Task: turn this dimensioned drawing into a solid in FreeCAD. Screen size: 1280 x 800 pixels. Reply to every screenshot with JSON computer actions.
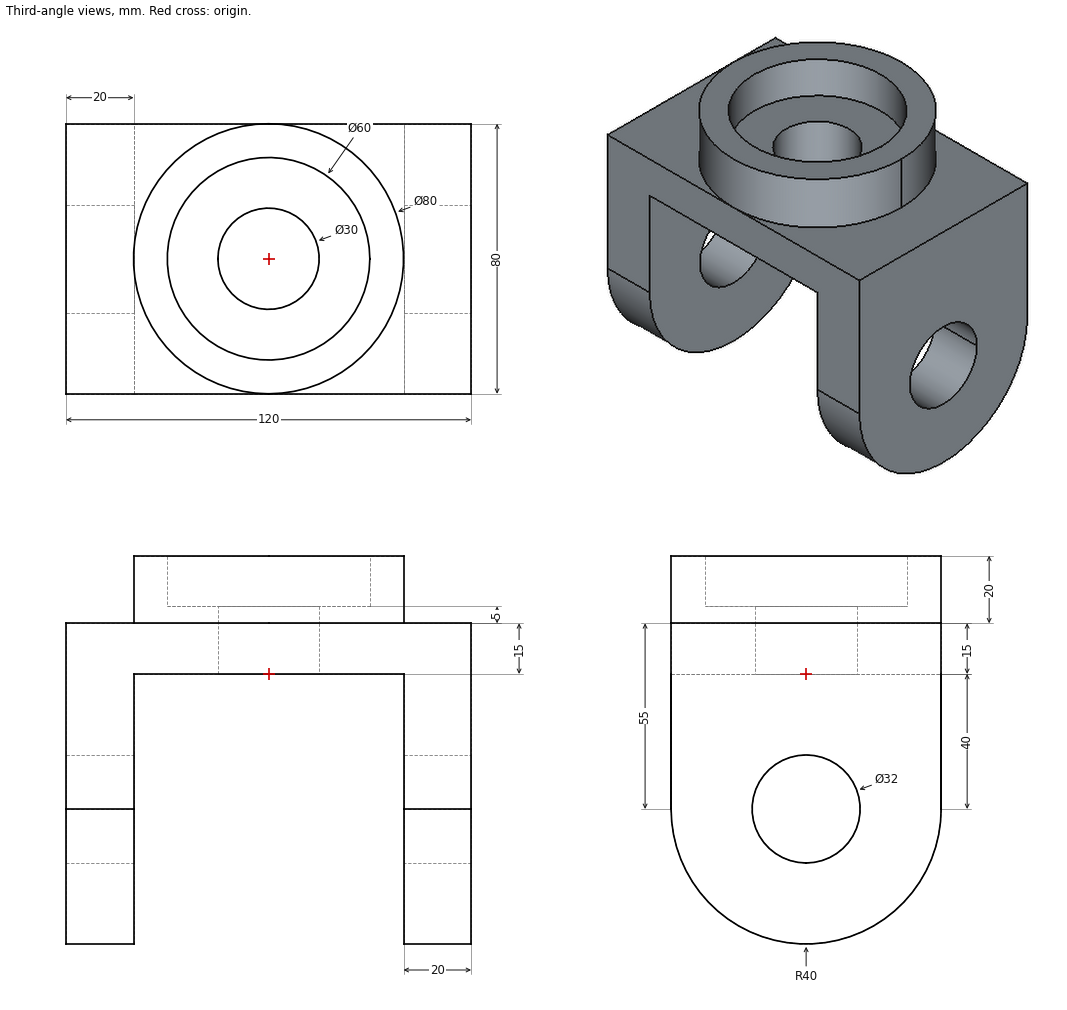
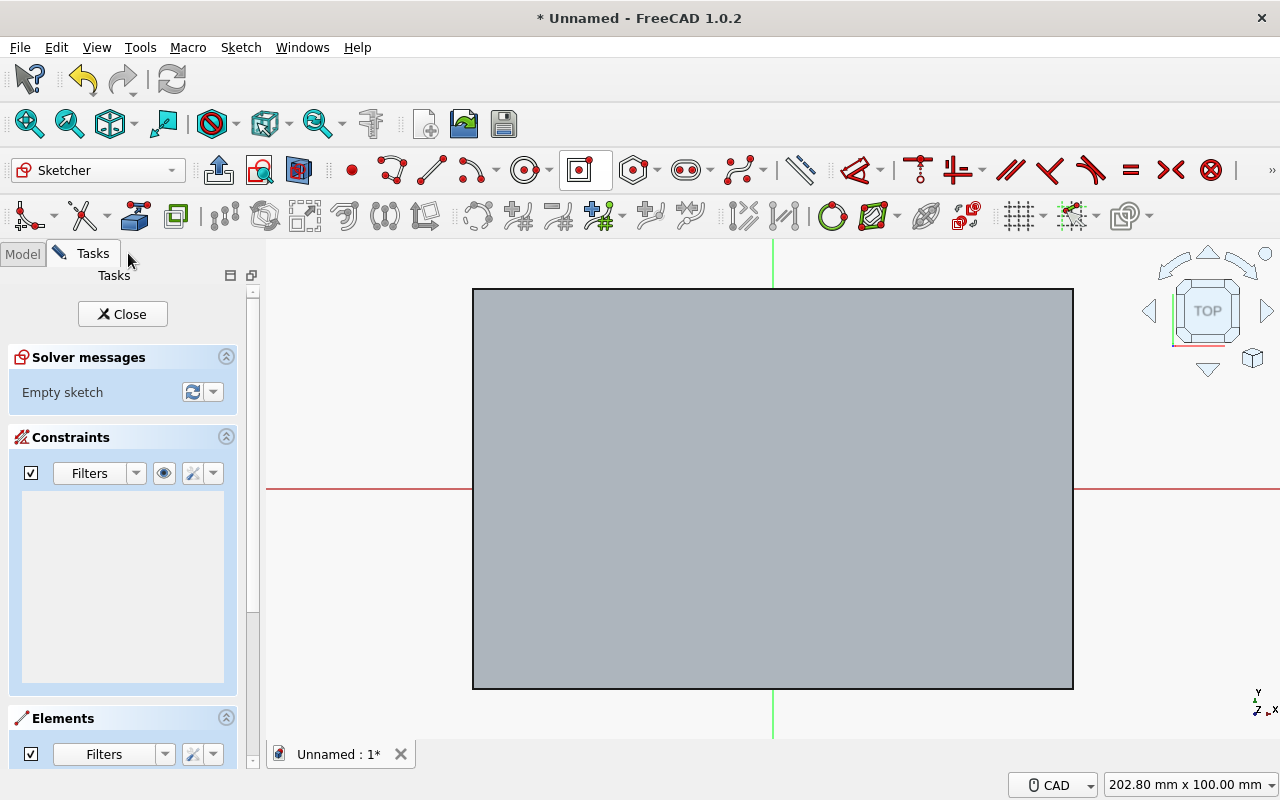
{"action": "key", "text": "q s"}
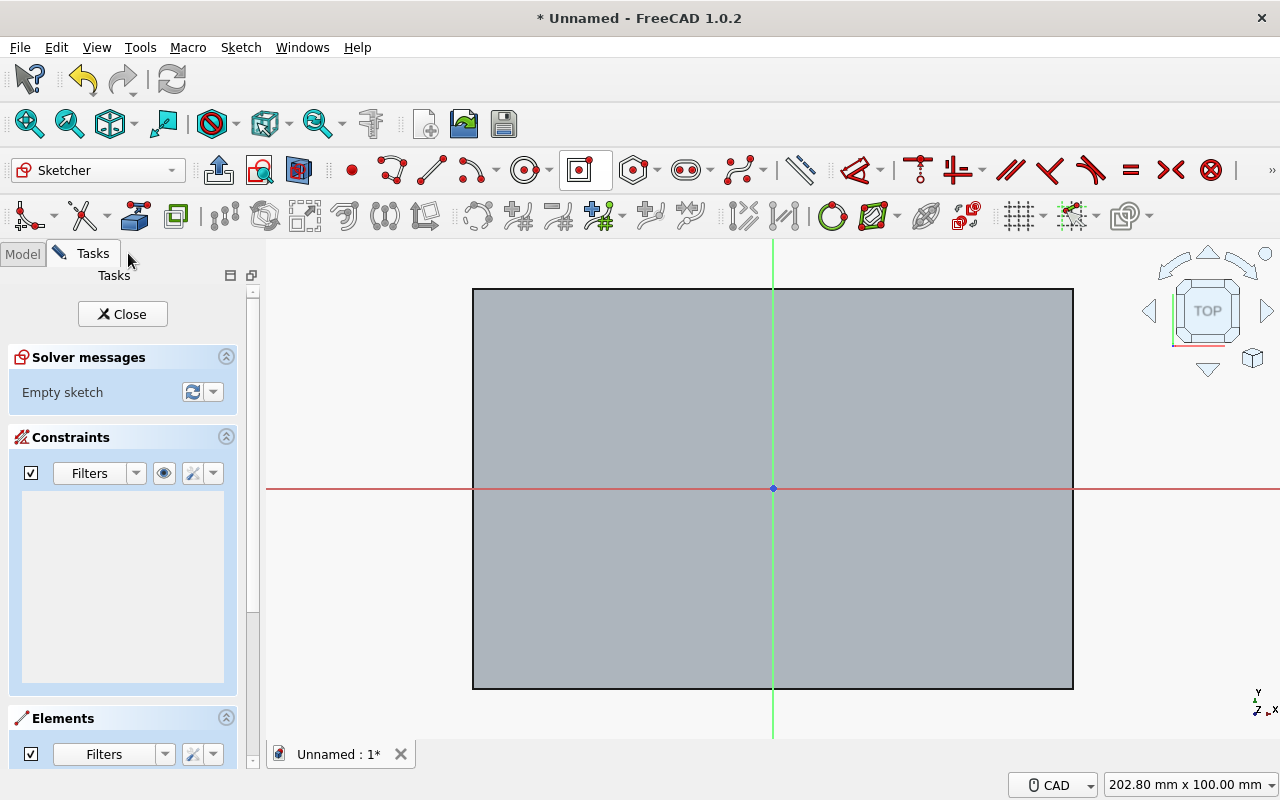
{"action": "scroll", "coordinate": [829, 489], "scroll_direction": "up", "scroll_amount": 4}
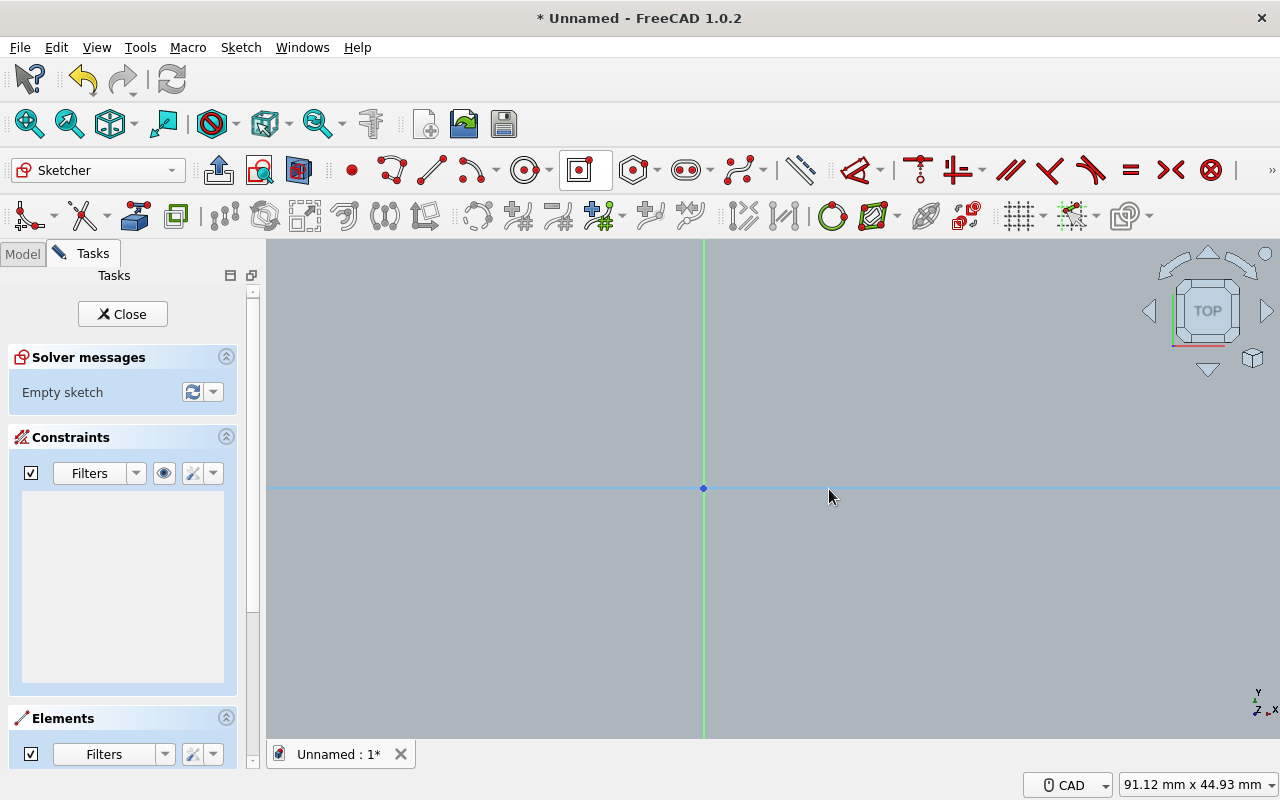
{"action": "left_click", "coordinate": [526, 170]}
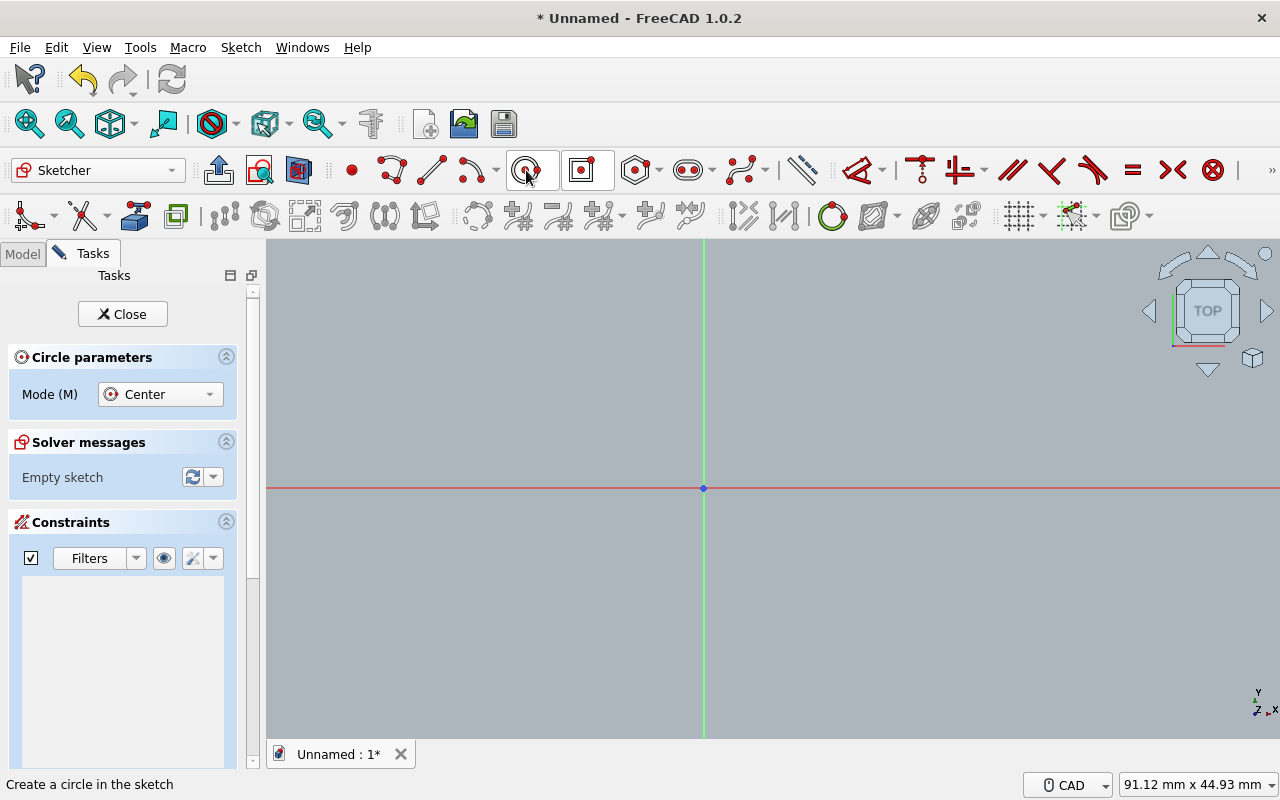
{"action": "left_click", "coordinate": [704, 488]}
{"action": "left_click", "coordinate": [822, 370]}
{"action": "key", "text": "Escape"}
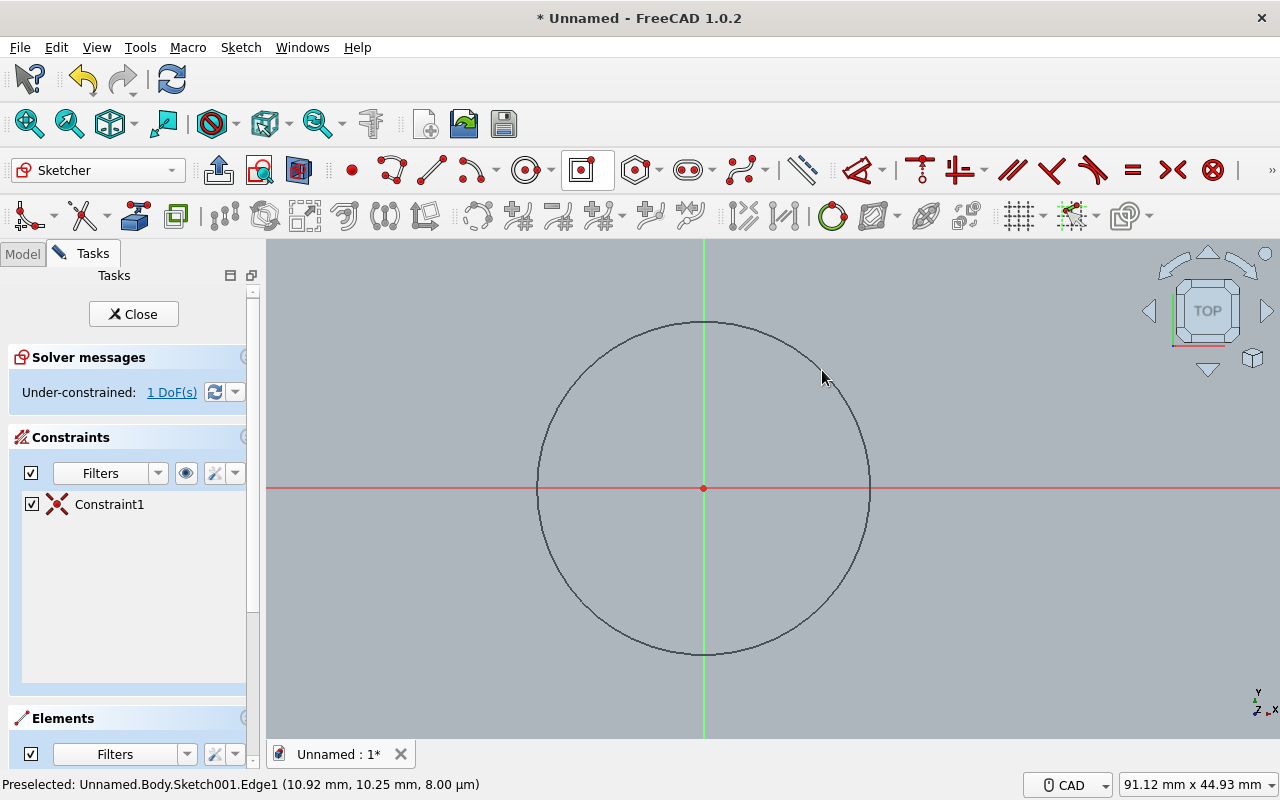
{"action": "left_click", "coordinate": [858, 170]}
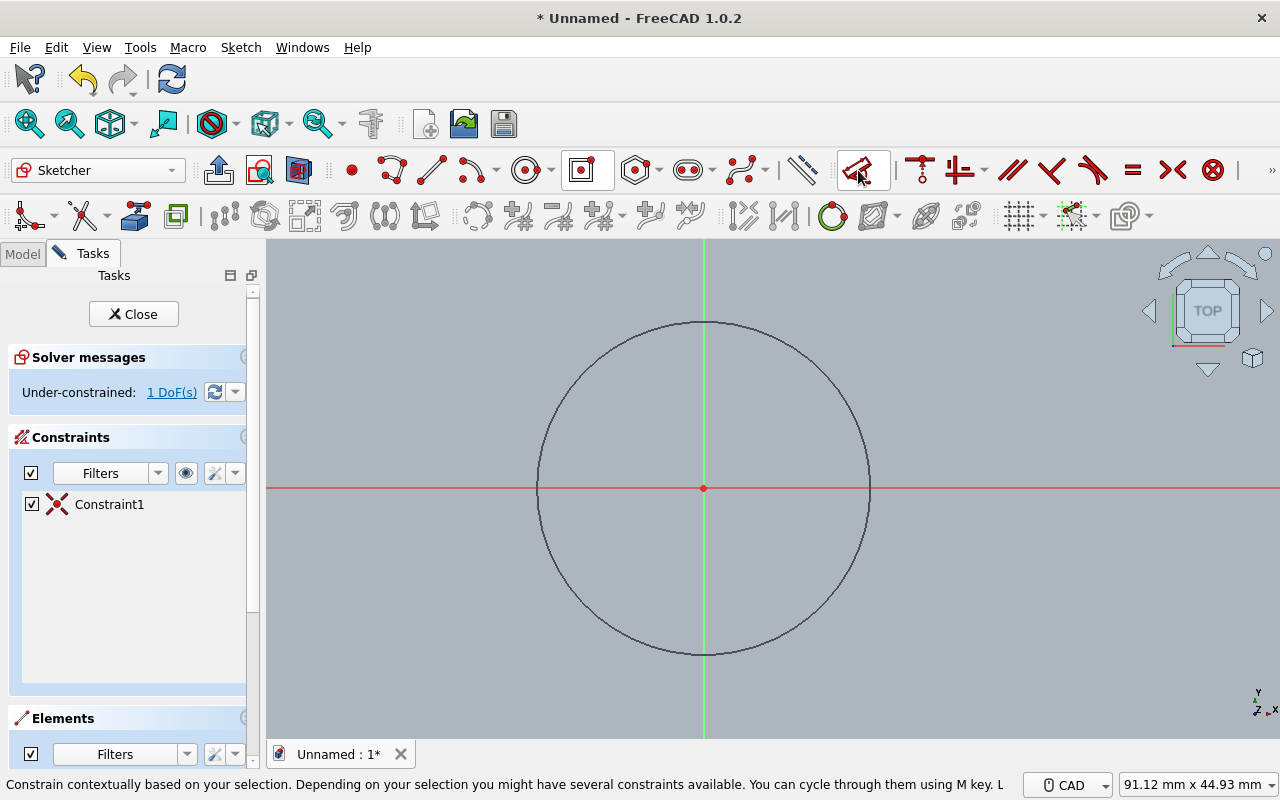
{"action": "left_click", "coordinate": [821, 370]}
{"action": "left_click", "coordinate": [844, 347]}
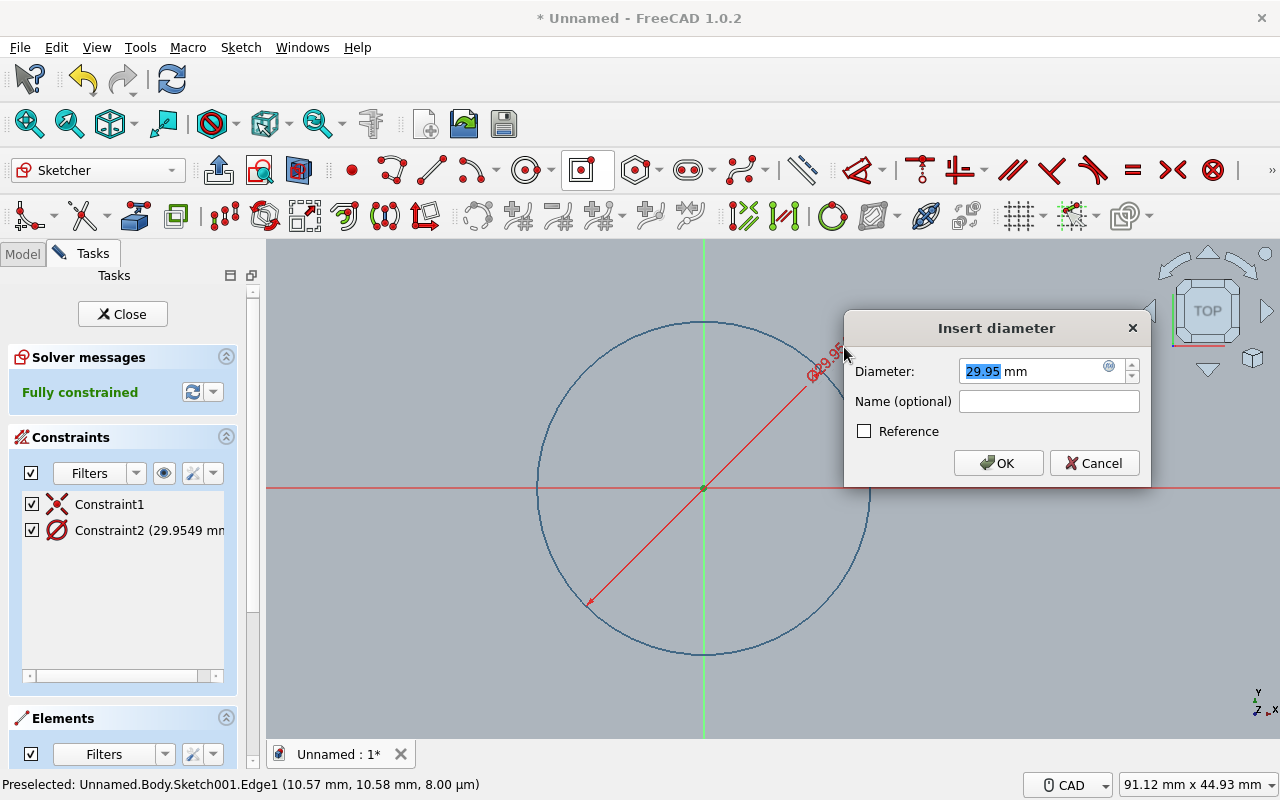
{"action": "type", "text": "30"}
{"action": "key", "text": "Return"}
{"action": "key", "text": "Escape"}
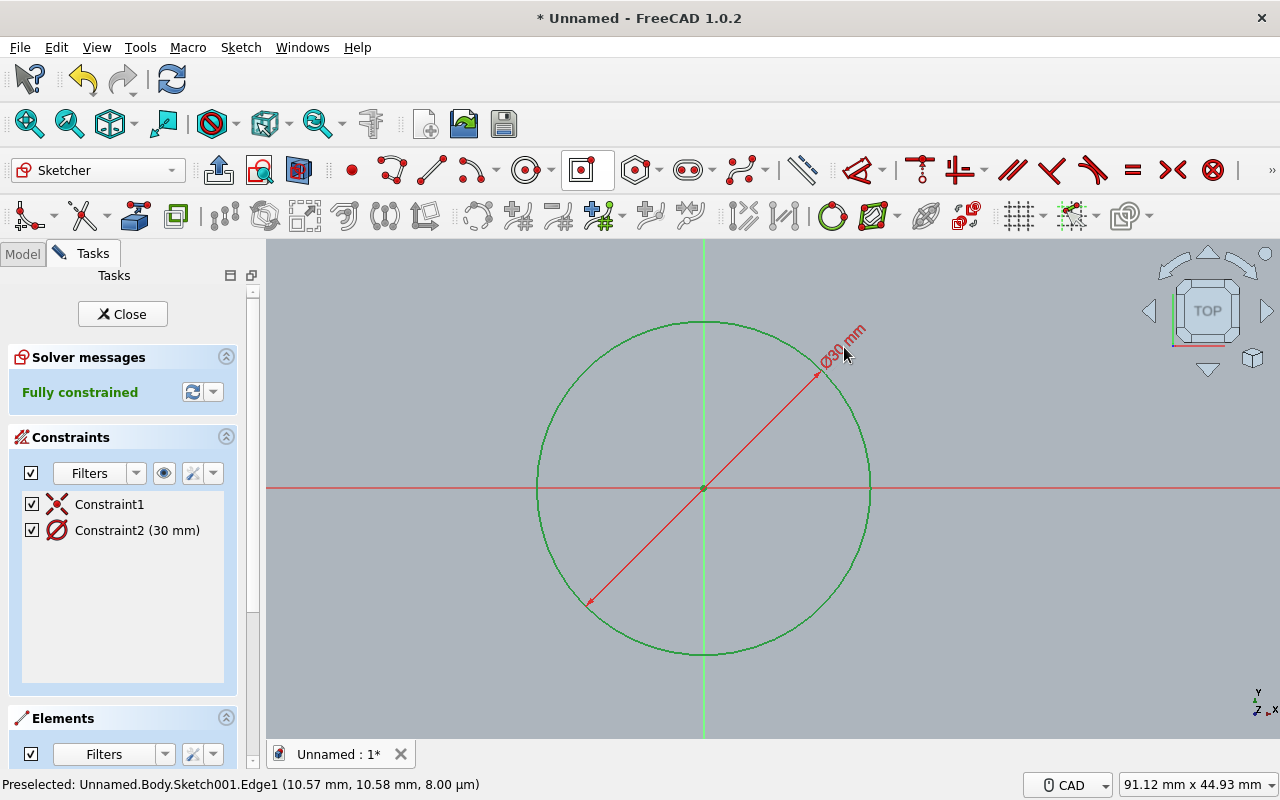
{"action": "left_click", "coordinate": [123, 314]}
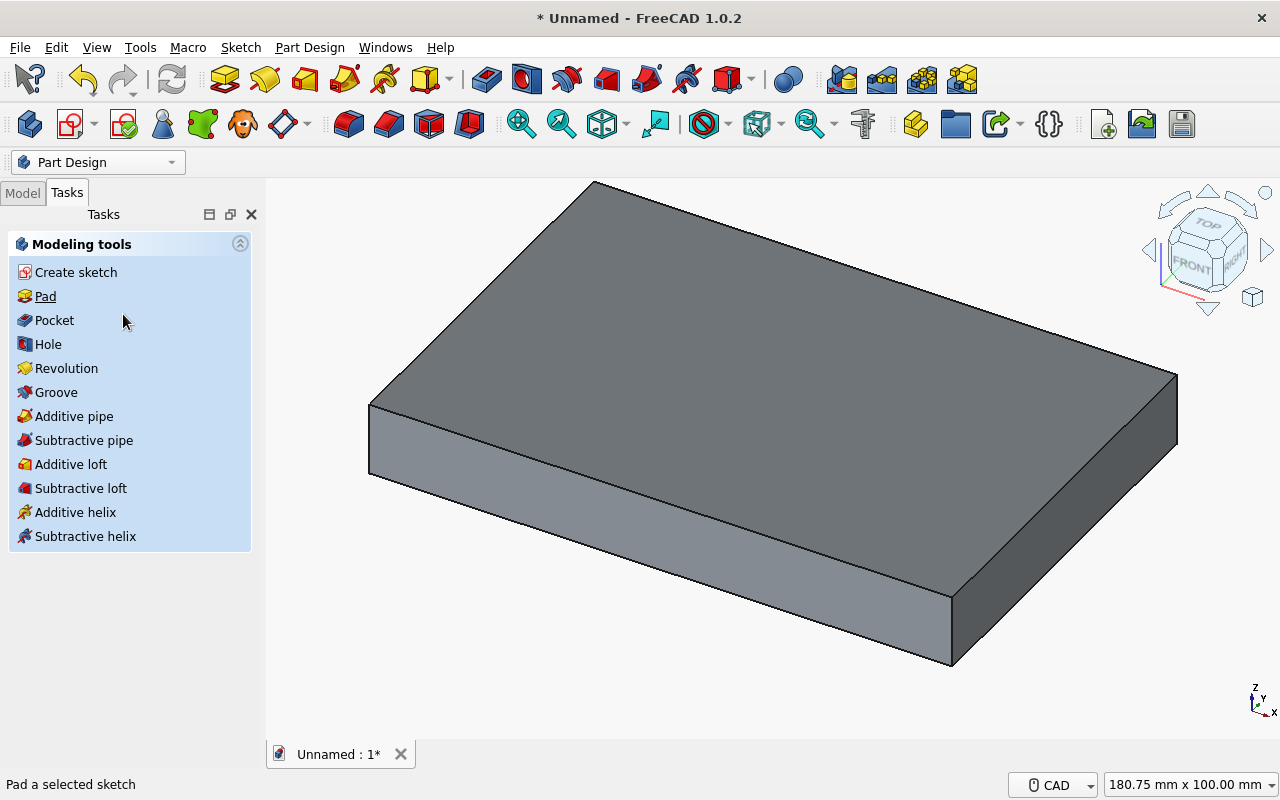
{"action": "left_click", "coordinate": [488, 80]}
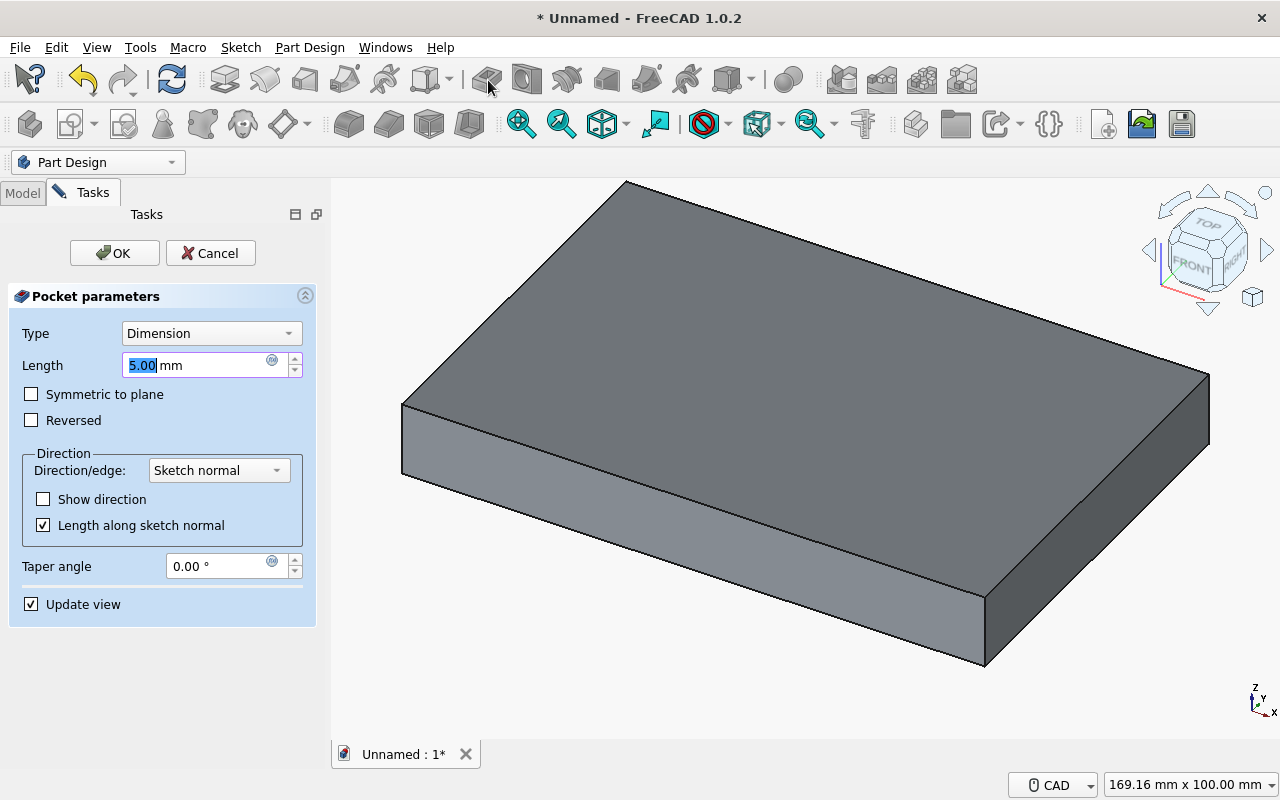
{"action": "type", "text": "15"}
{"action": "key", "text": "Tab"}